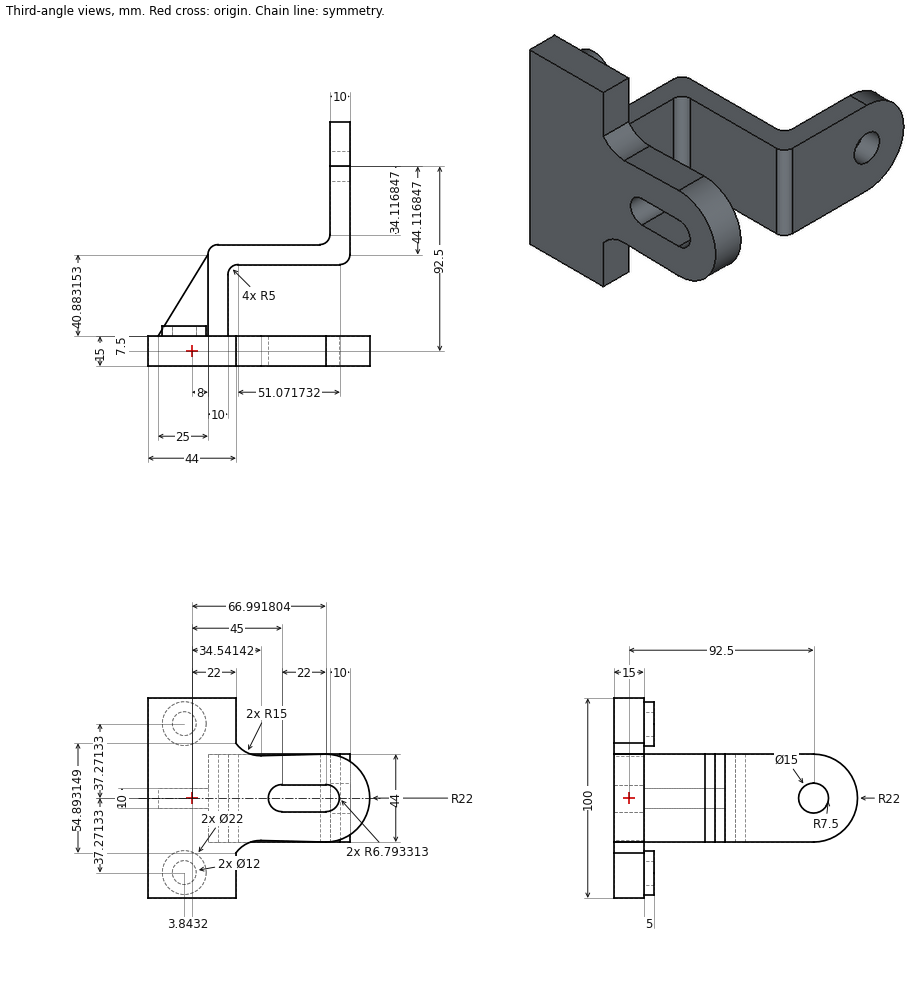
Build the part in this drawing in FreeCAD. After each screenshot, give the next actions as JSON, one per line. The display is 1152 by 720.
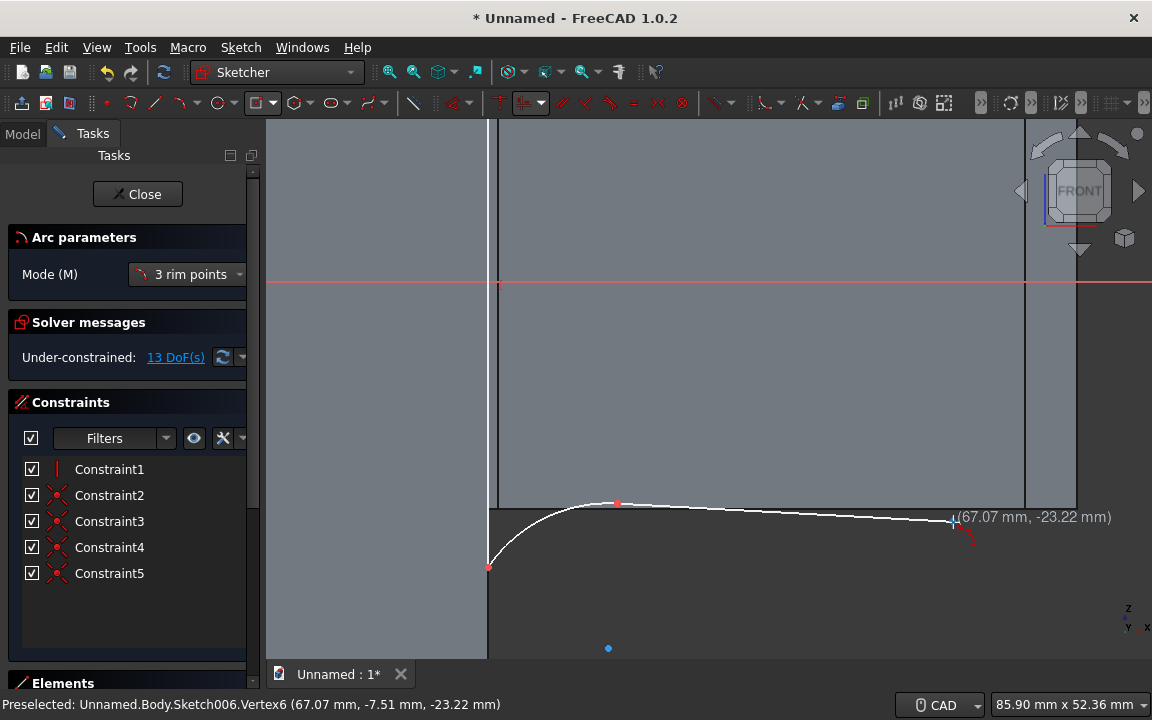
{"action": "scroll", "coordinate": [544, 519], "scroll_direction": "down", "scroll_amount": 3}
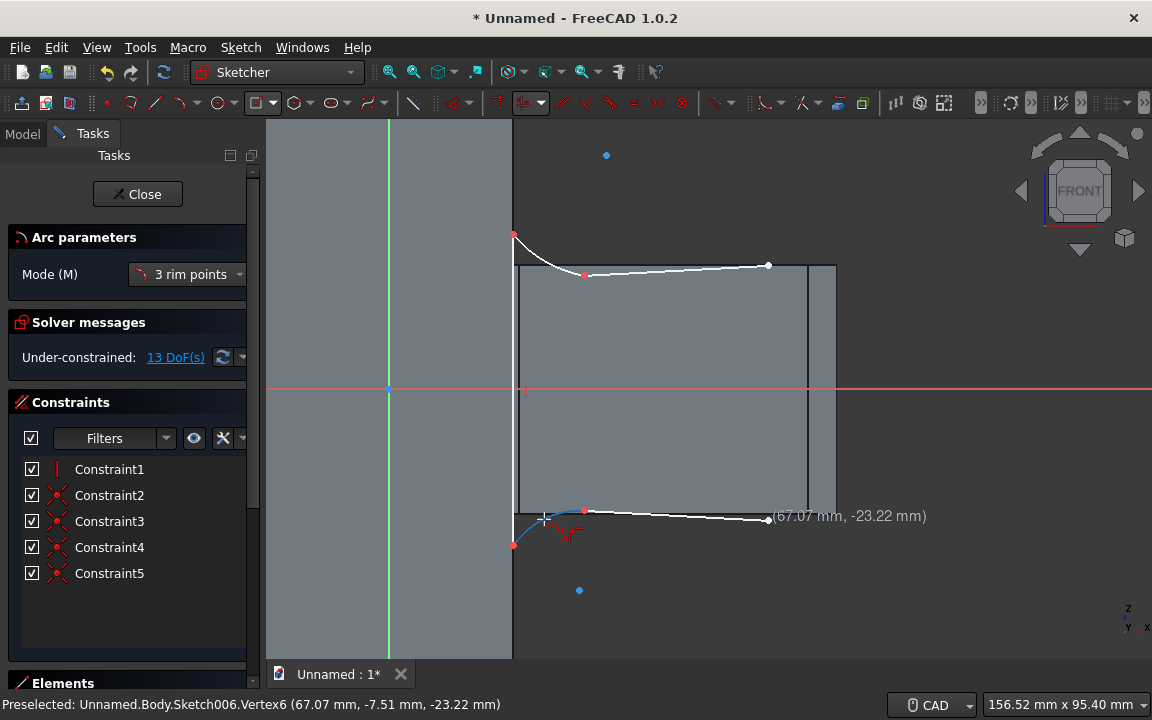
{"action": "left_click", "coordinate": [768, 266]}
{"action": "left_click", "coordinate": [886, 428]}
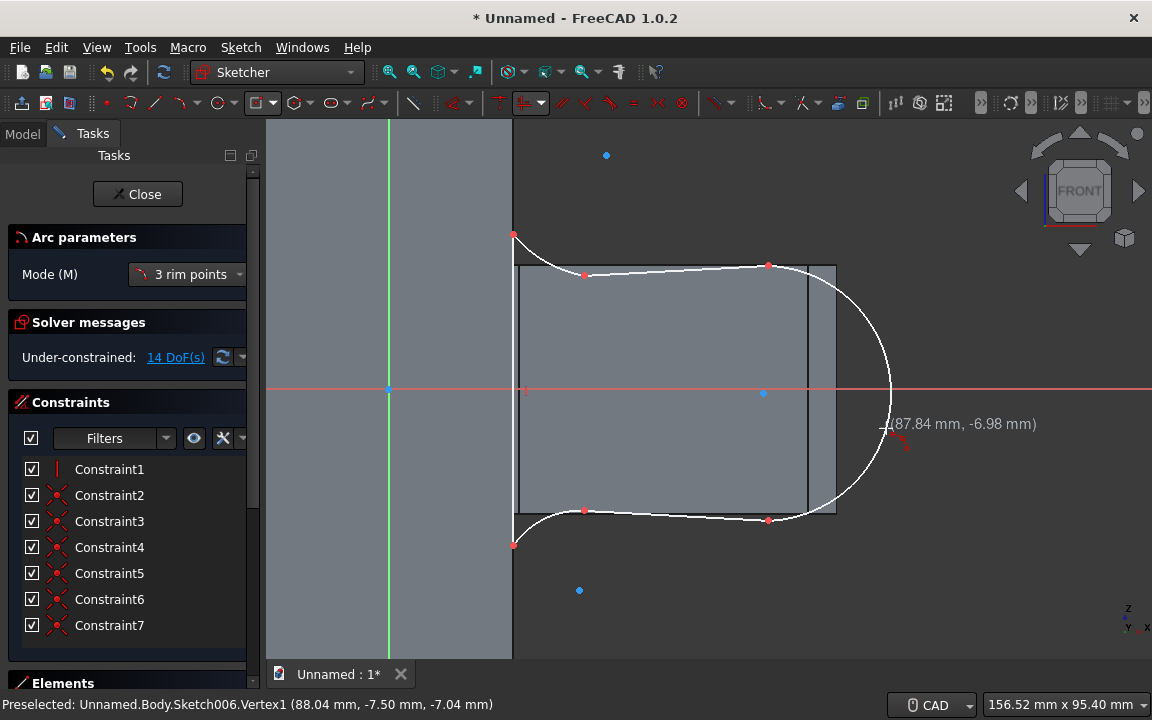
{"action": "left_click", "coordinate": [332, 104]}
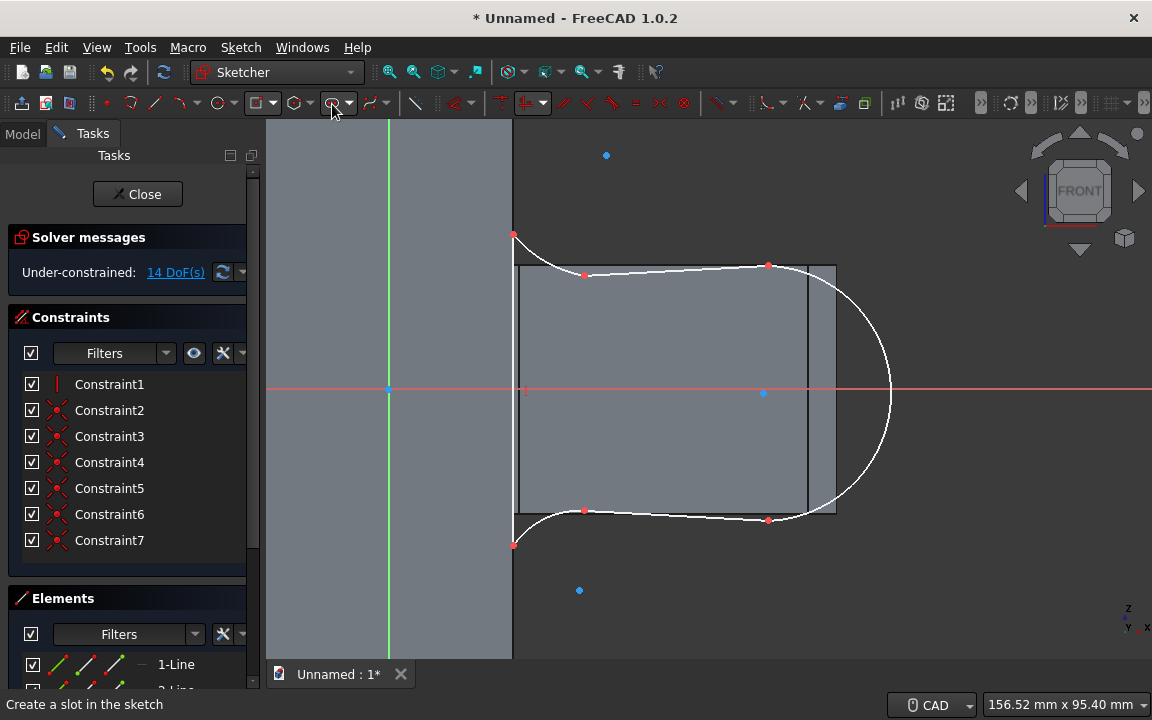
{"action": "left_click", "coordinate": [644, 389]}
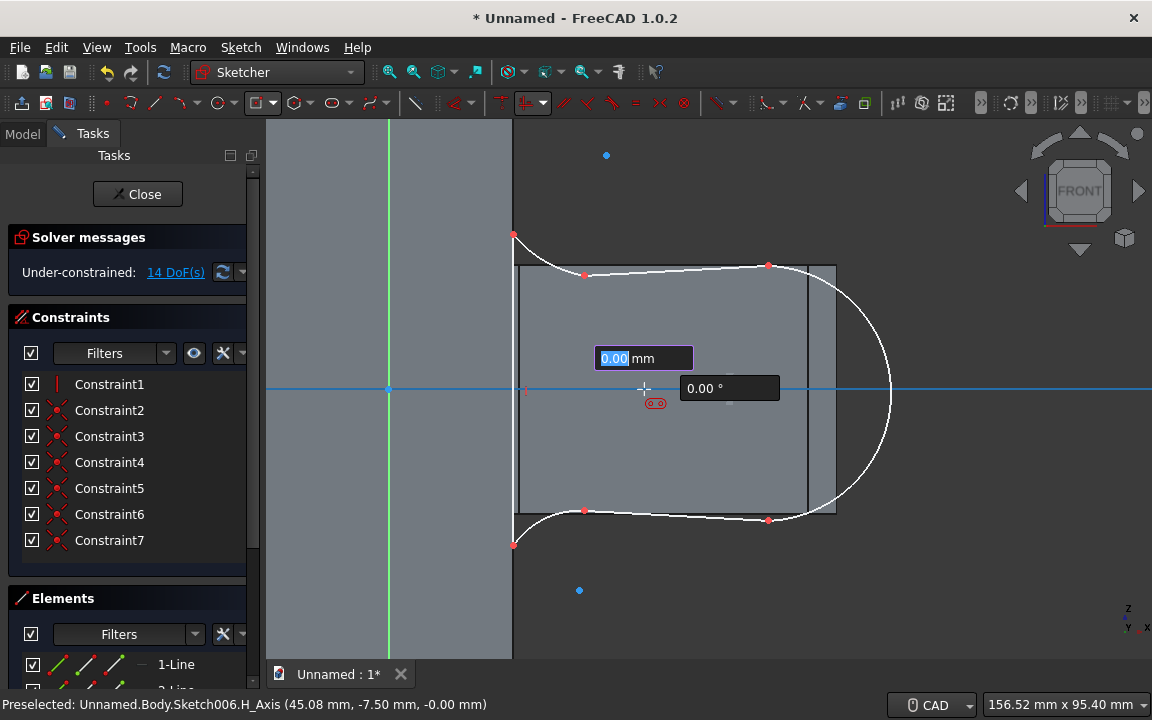
{"action": "left_click", "coordinate": [768, 380]}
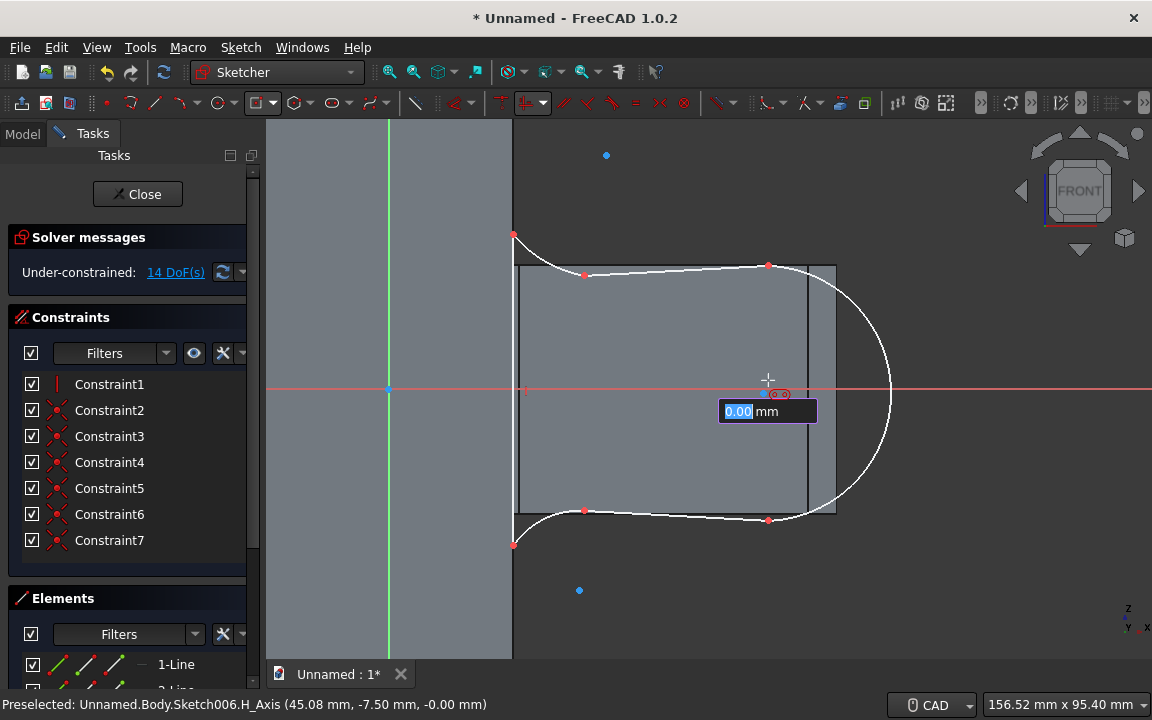
{"action": "left_click", "coordinate": [706, 351]}
{"action": "key", "text": "Escape"}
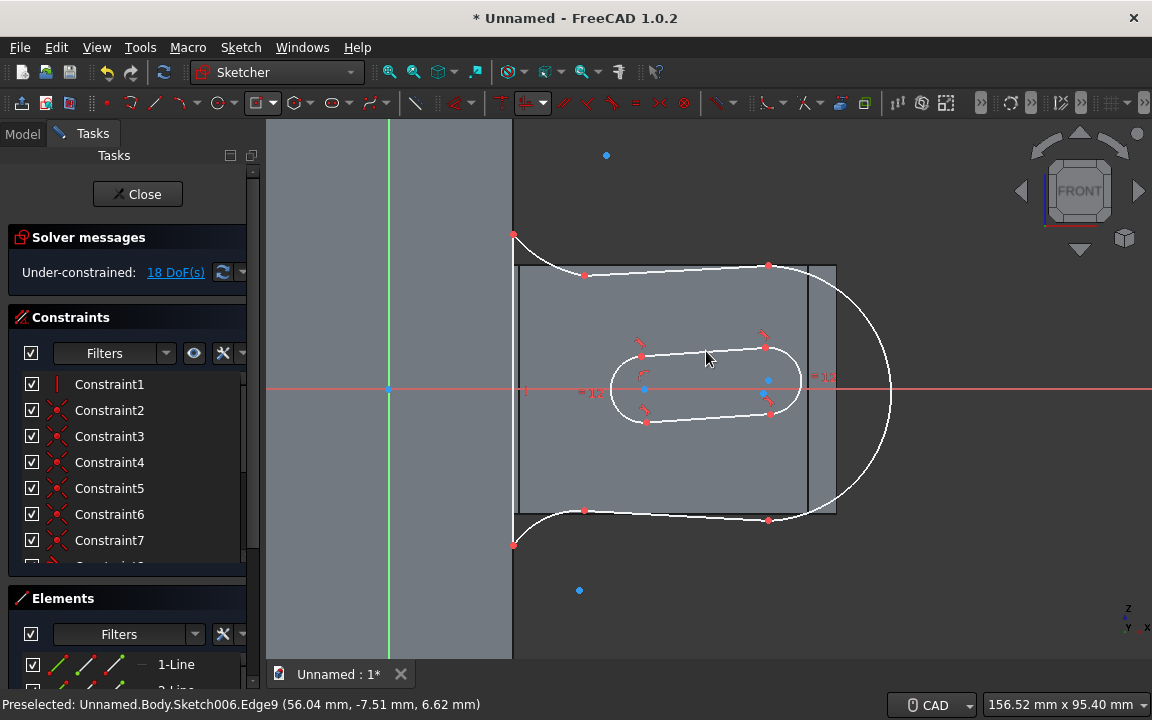
{"action": "left_click", "coordinate": [713, 269]}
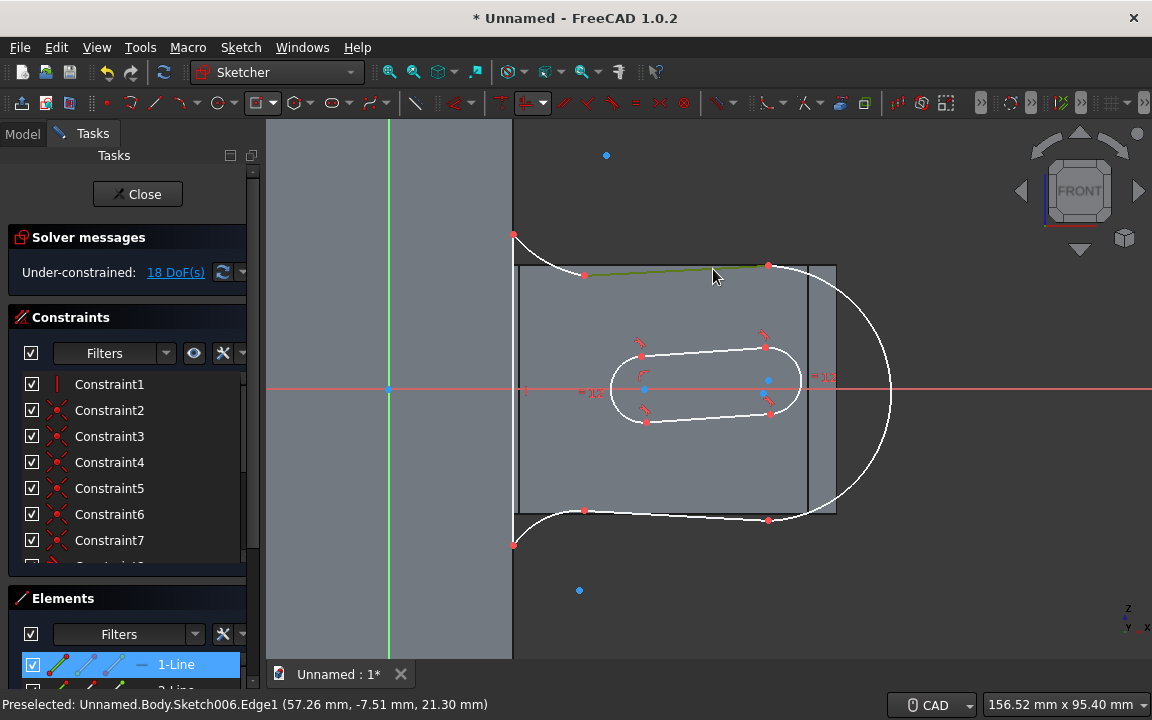
{"action": "left_click", "coordinate": [532, 252]}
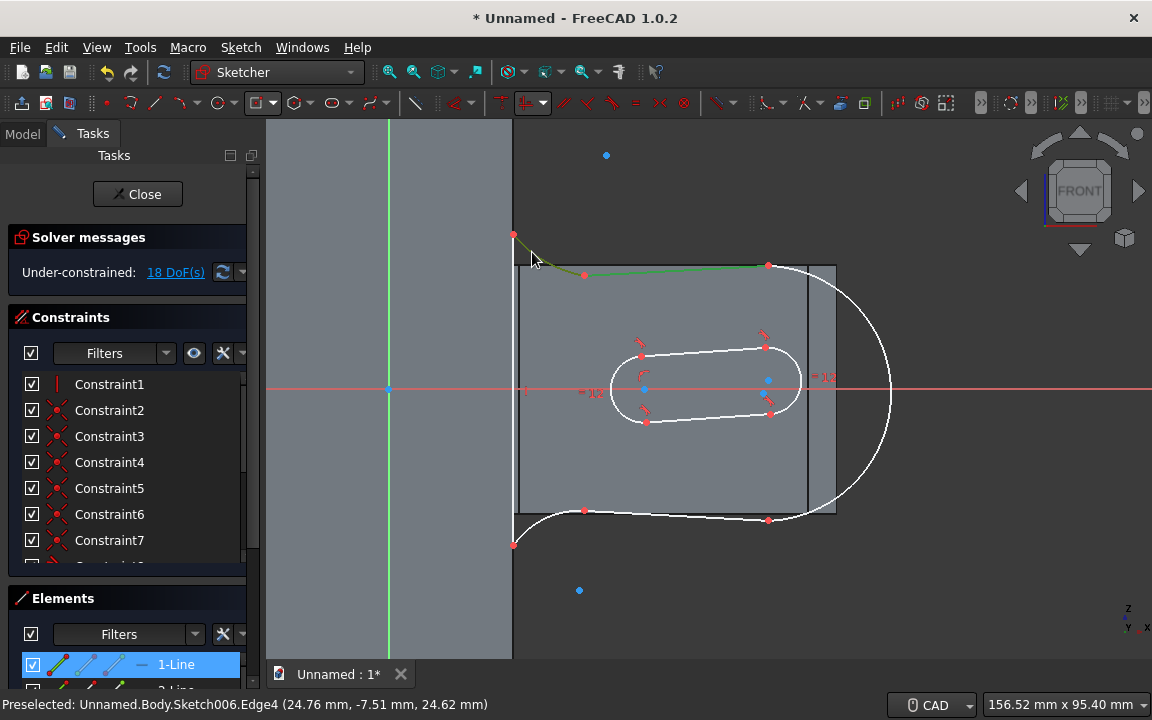
{"action": "left_click", "coordinate": [612, 104]}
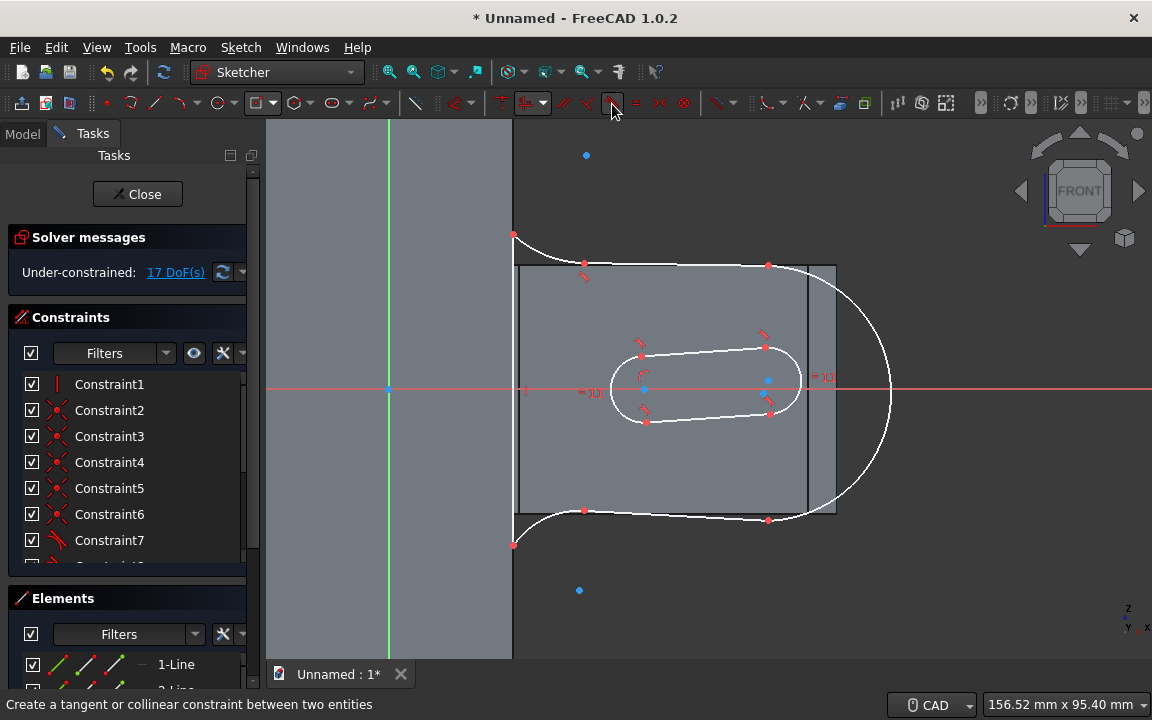
{"action": "left_click", "coordinate": [640, 514]}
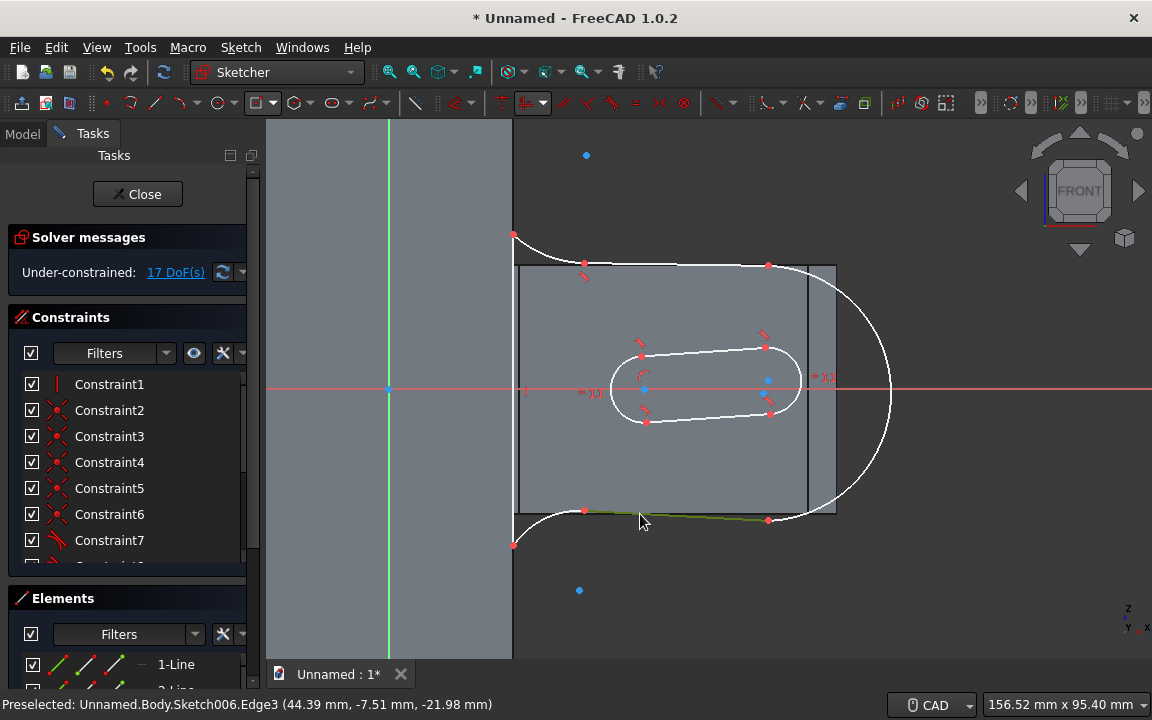
{"action": "left_click", "coordinate": [560, 513]}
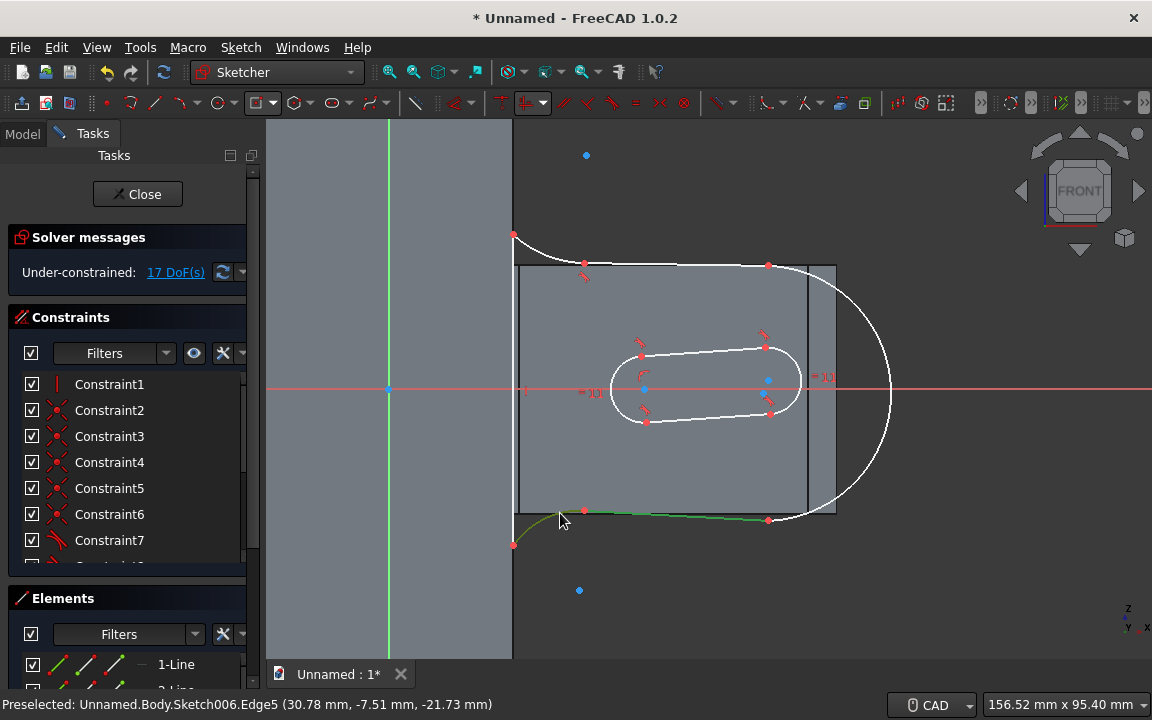
{"action": "left_click", "coordinate": [612, 104]}